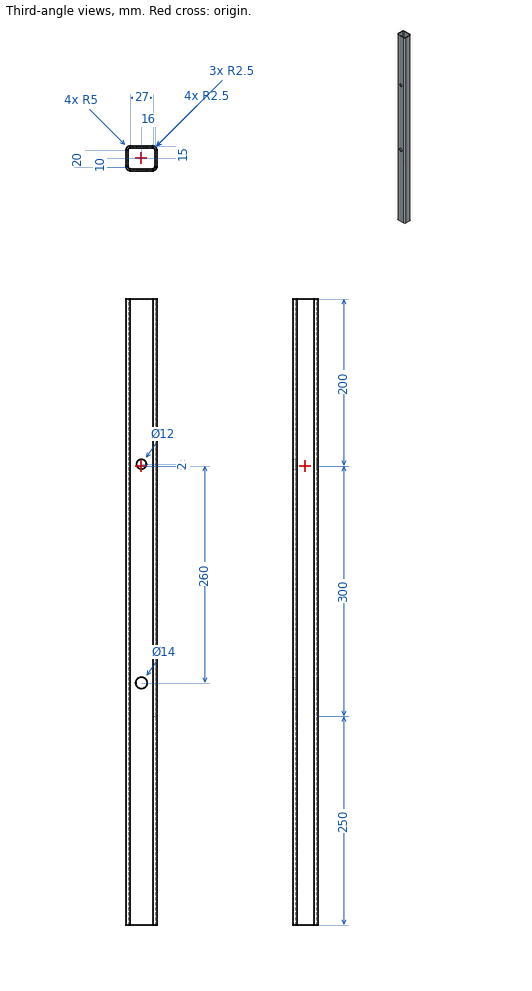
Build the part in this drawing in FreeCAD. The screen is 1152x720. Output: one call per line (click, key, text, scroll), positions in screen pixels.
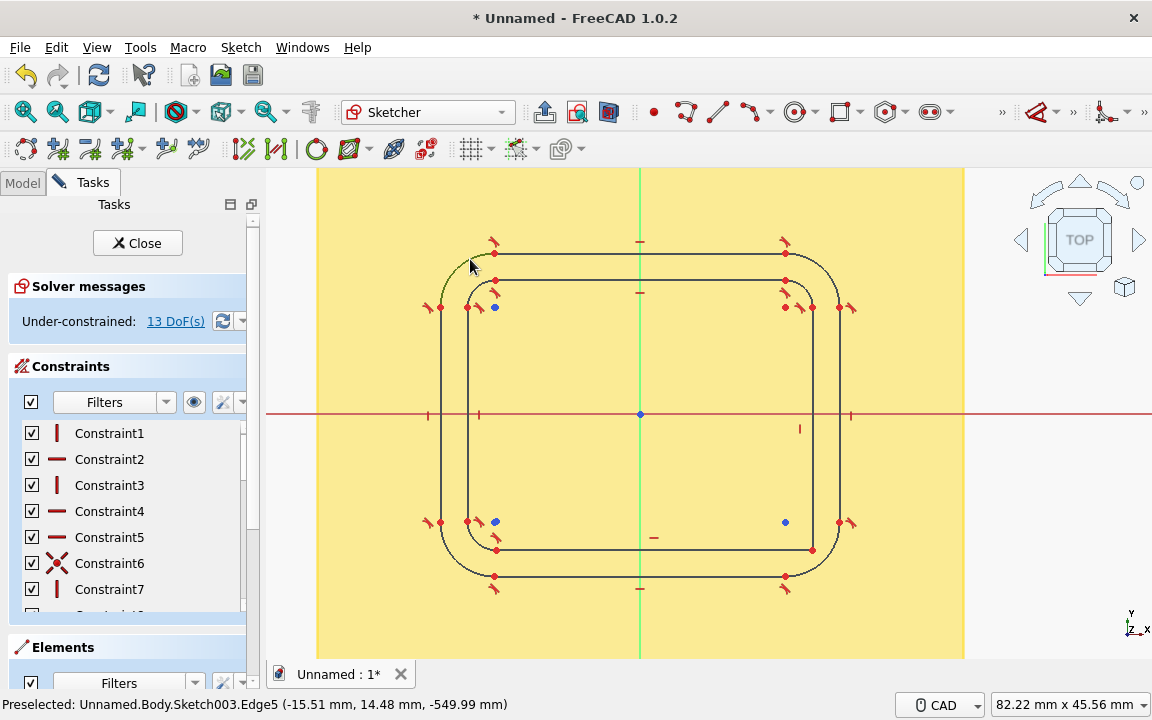
click(483, 283)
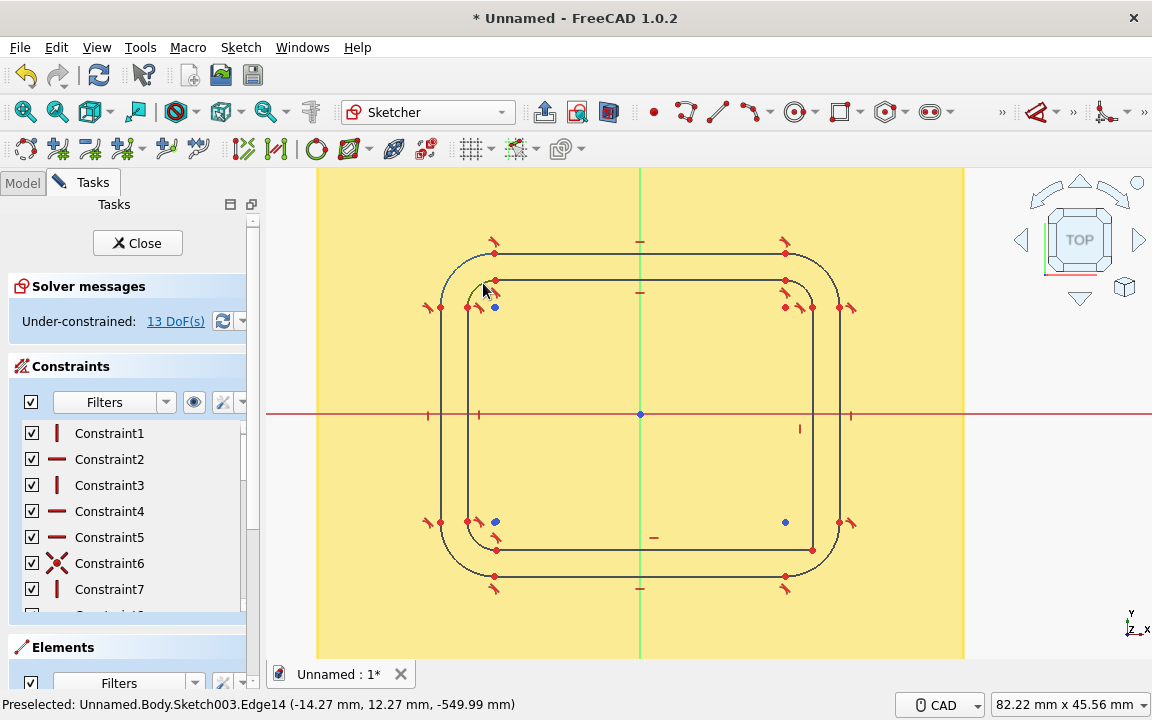
key(c)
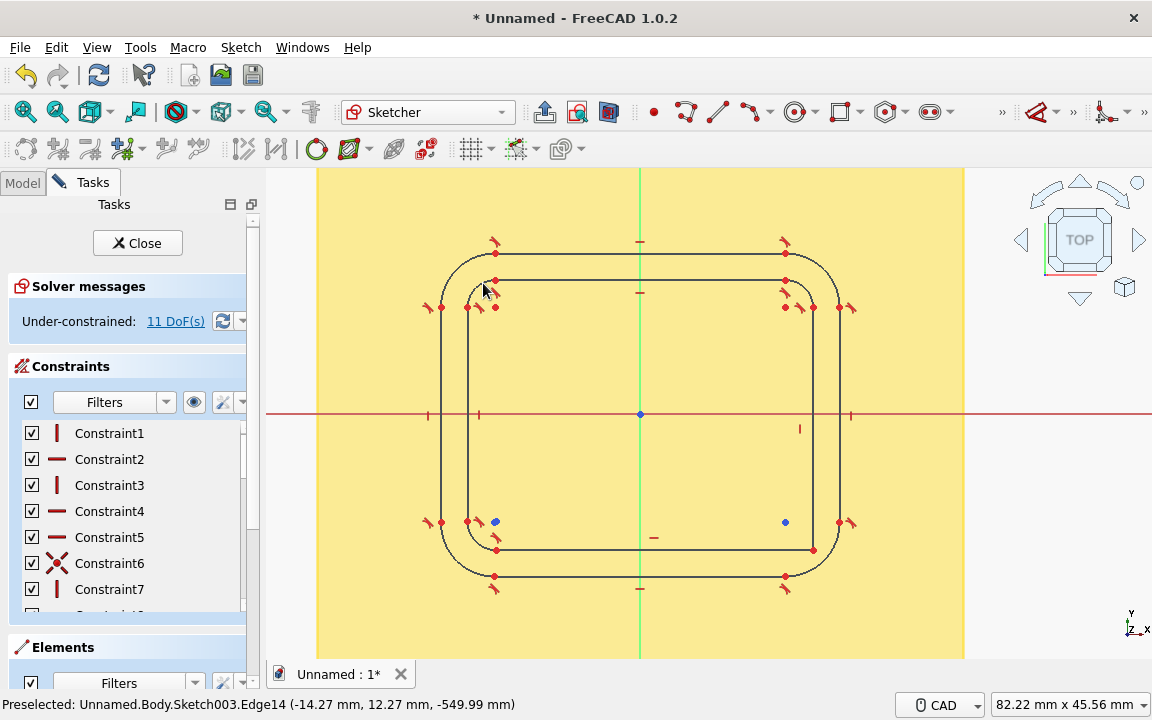
click(447, 547)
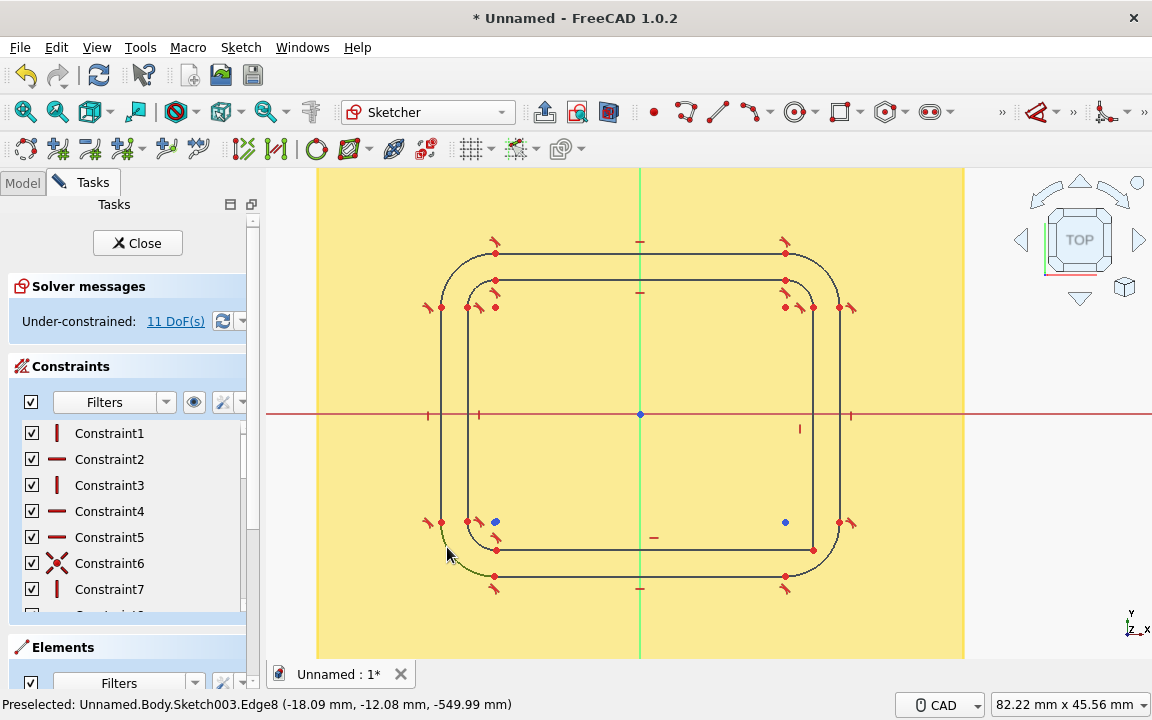
click(471, 534)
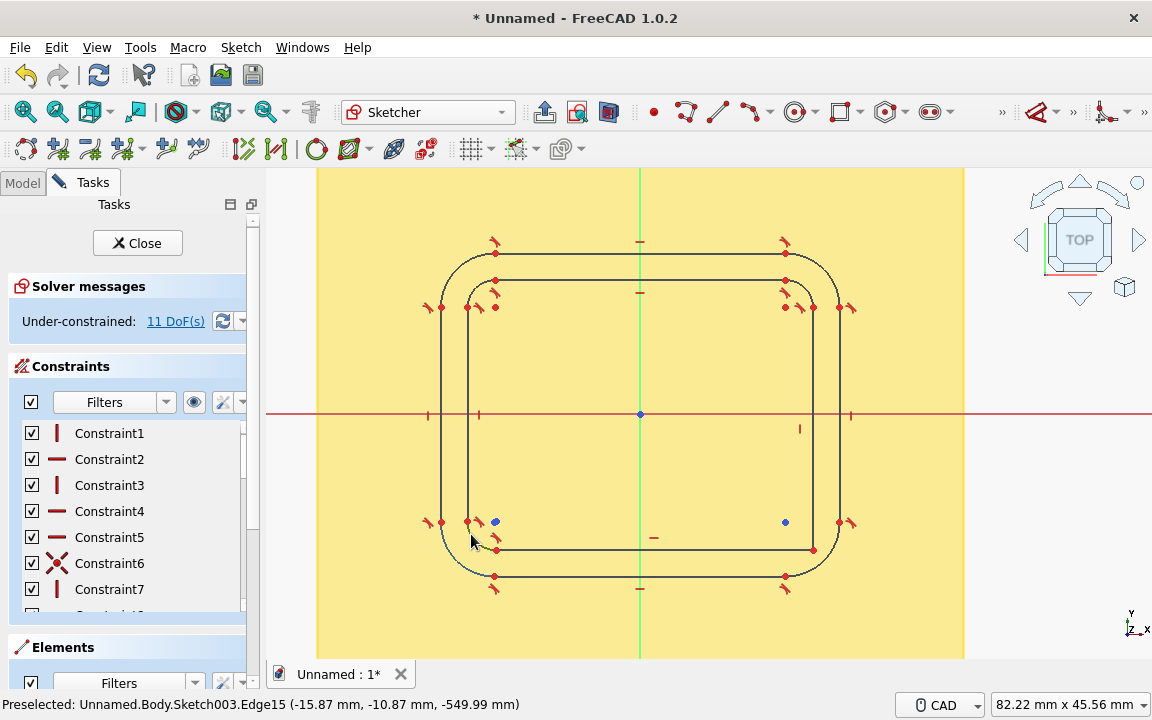
key(c)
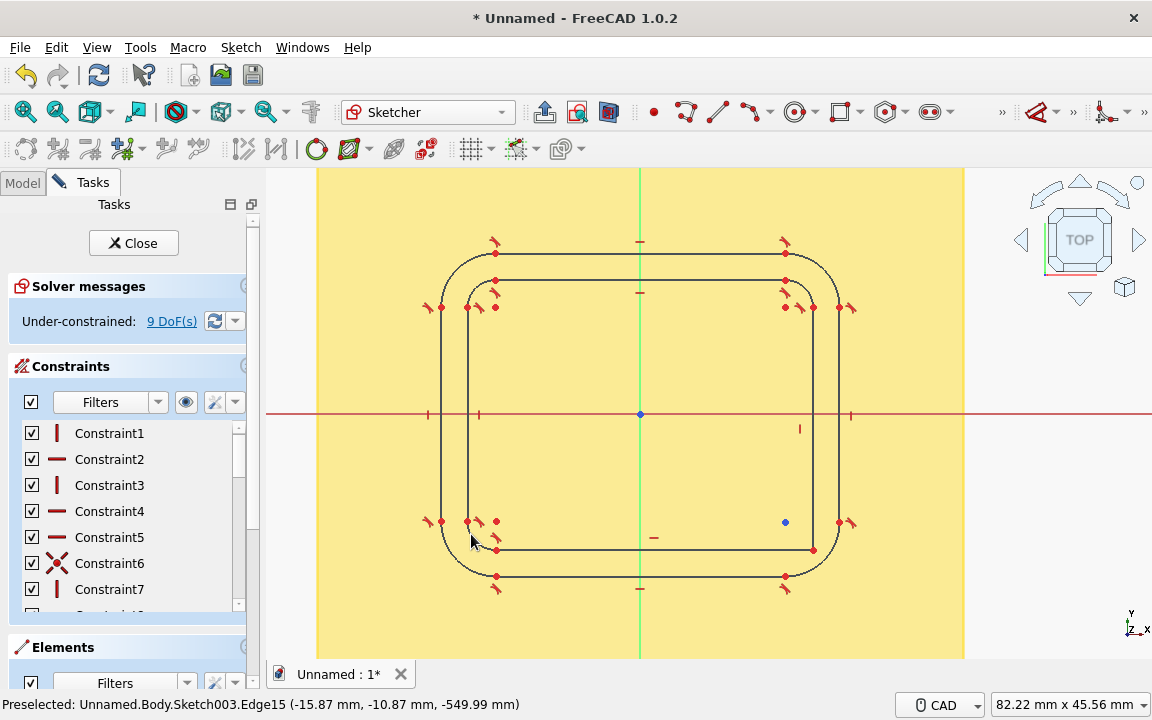
click(471, 260)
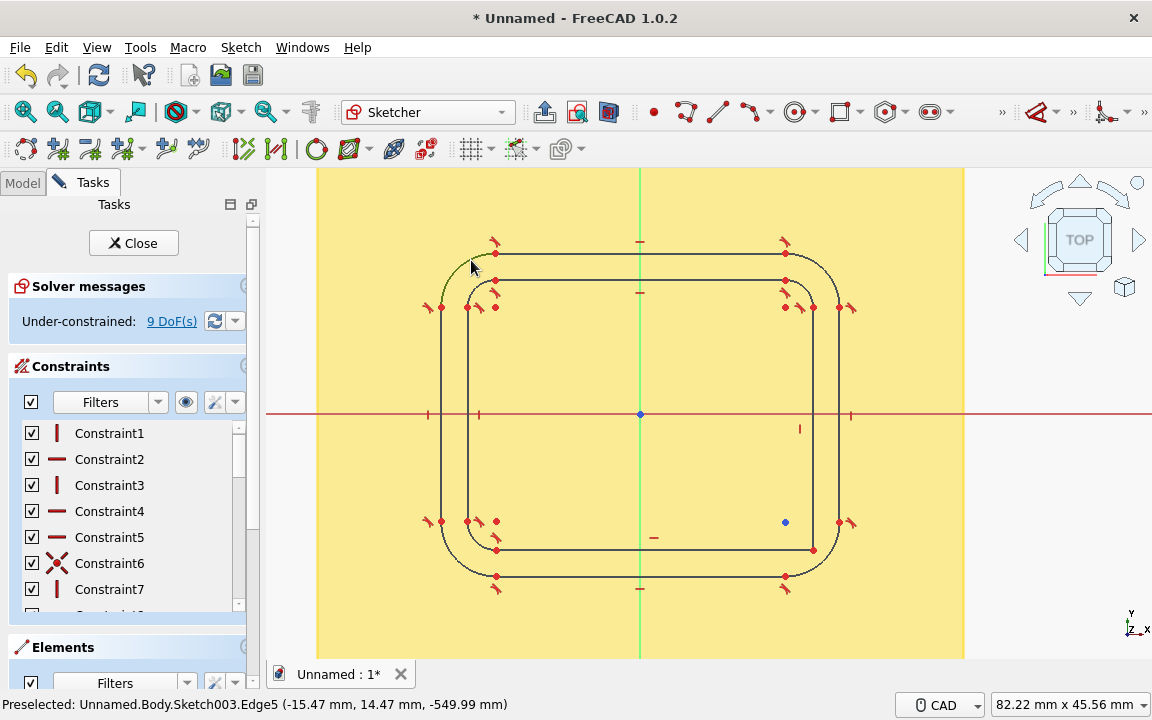
click(834, 283)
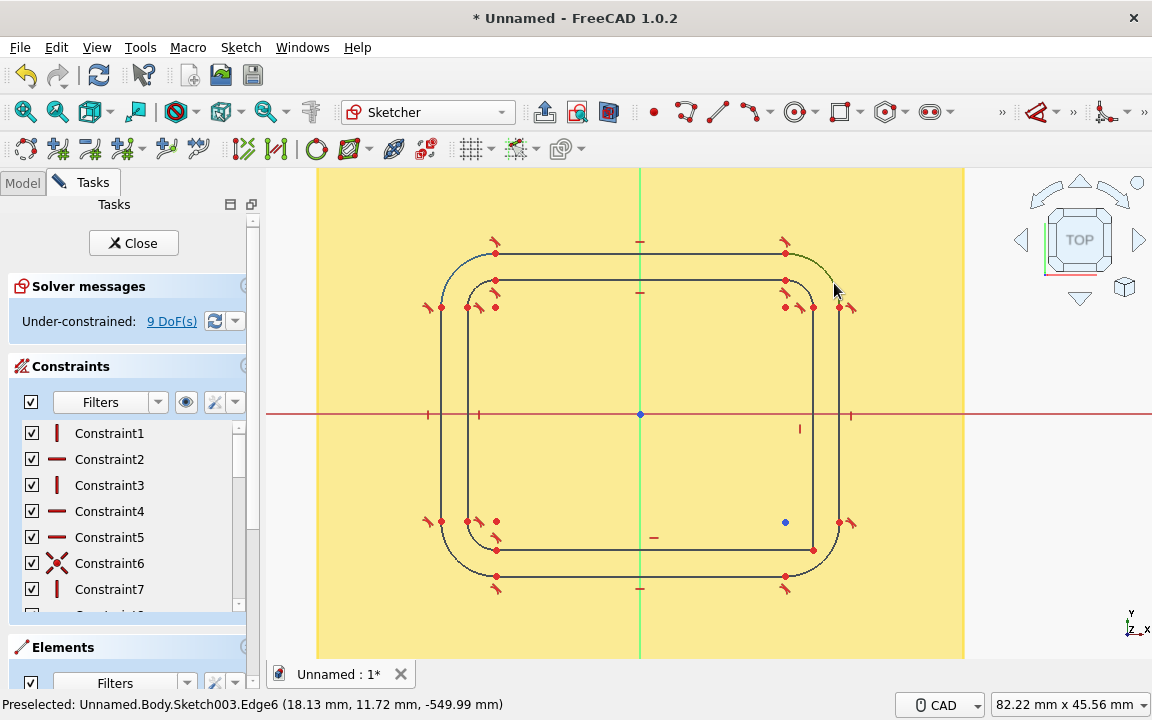
click(810, 571)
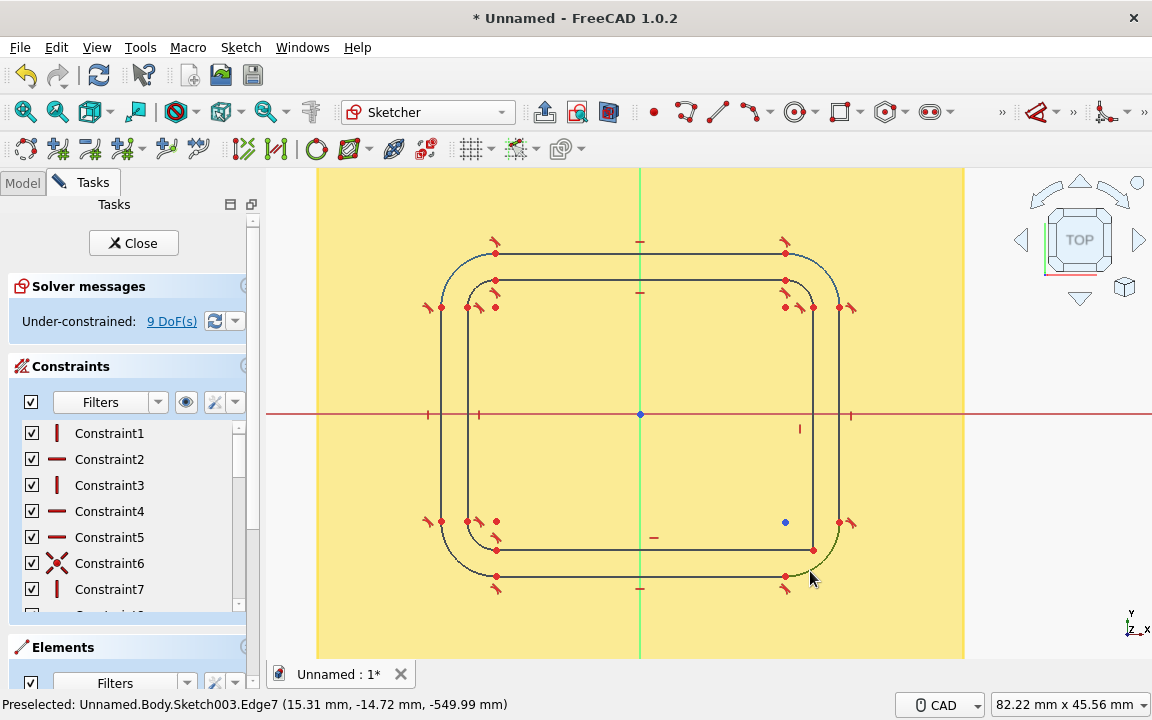
click(447, 546)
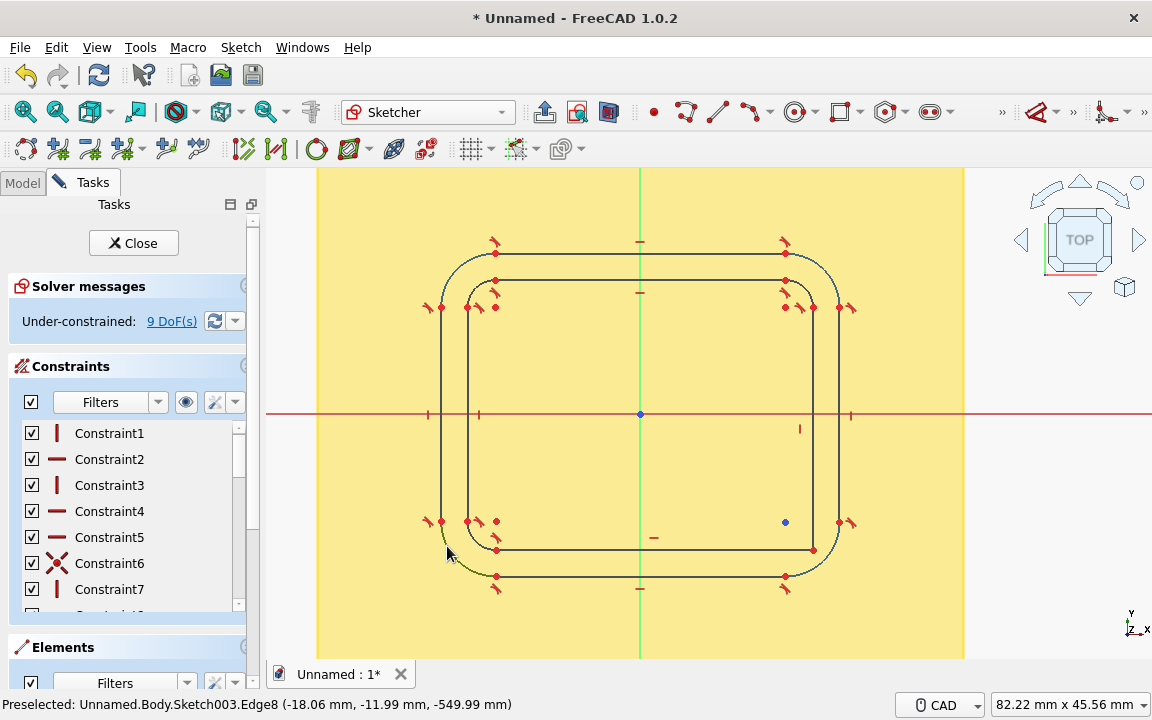
key(e)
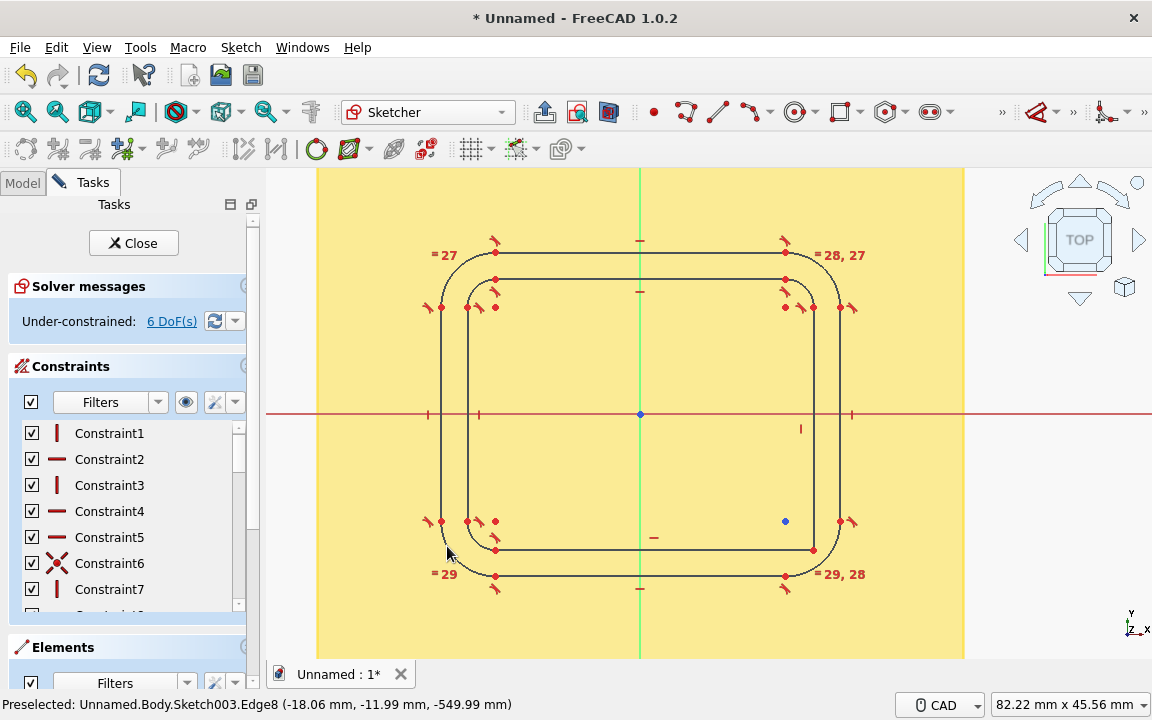
key(d)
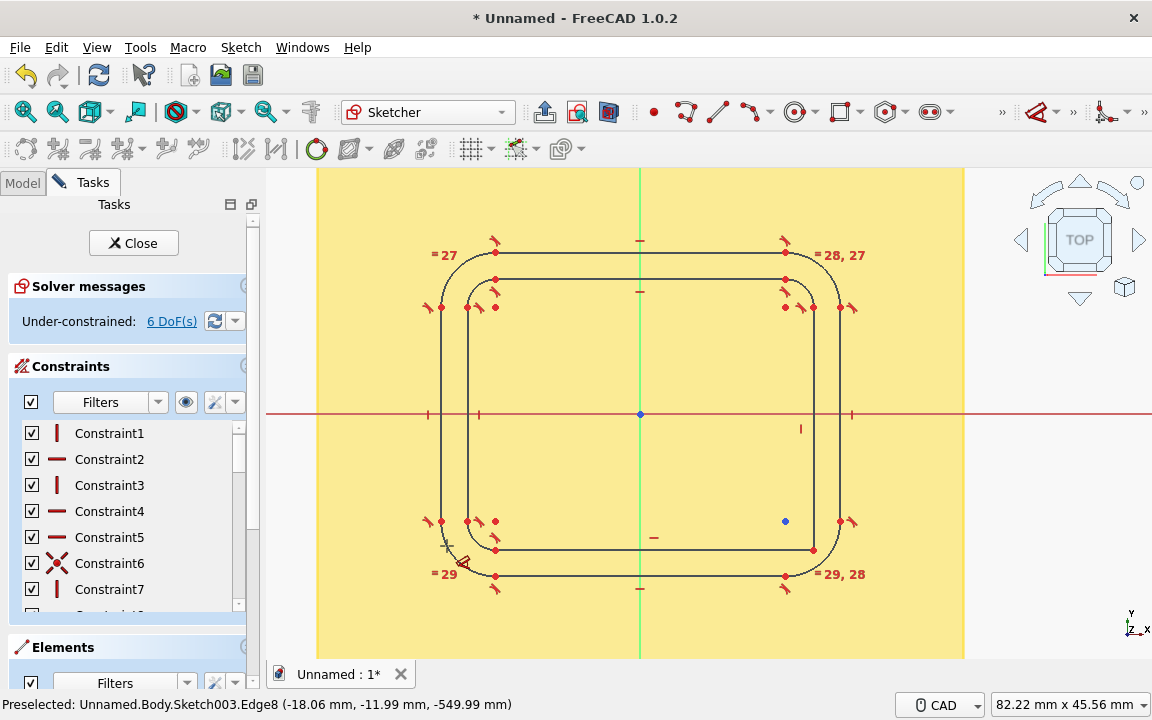
click(471, 259)
click(456, 231)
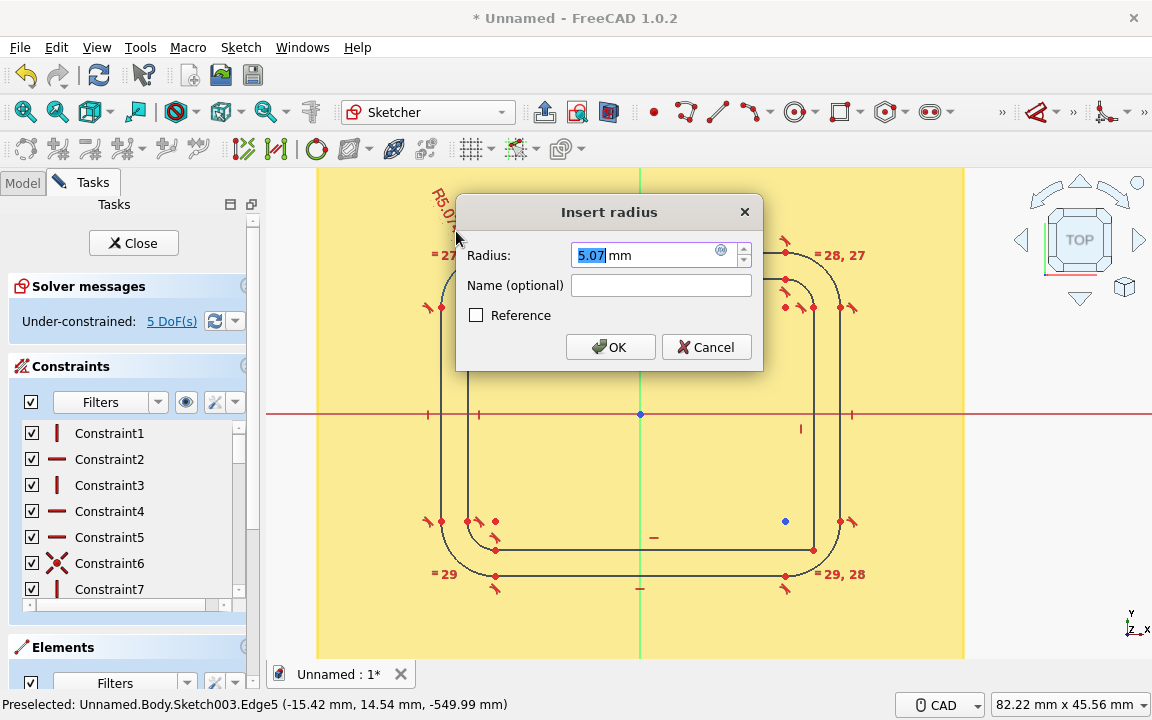
text(5)
key(Return)